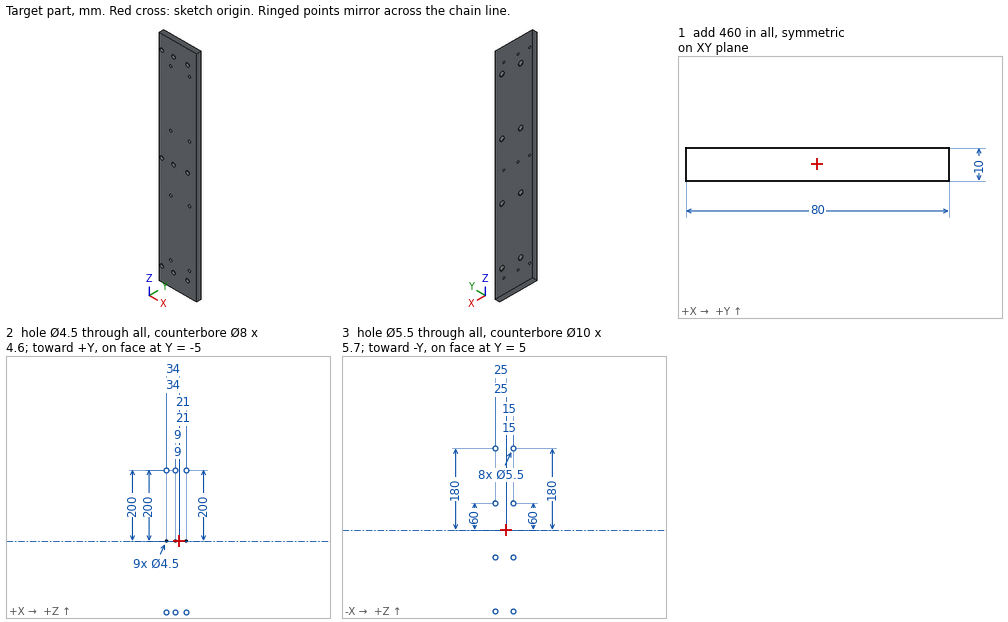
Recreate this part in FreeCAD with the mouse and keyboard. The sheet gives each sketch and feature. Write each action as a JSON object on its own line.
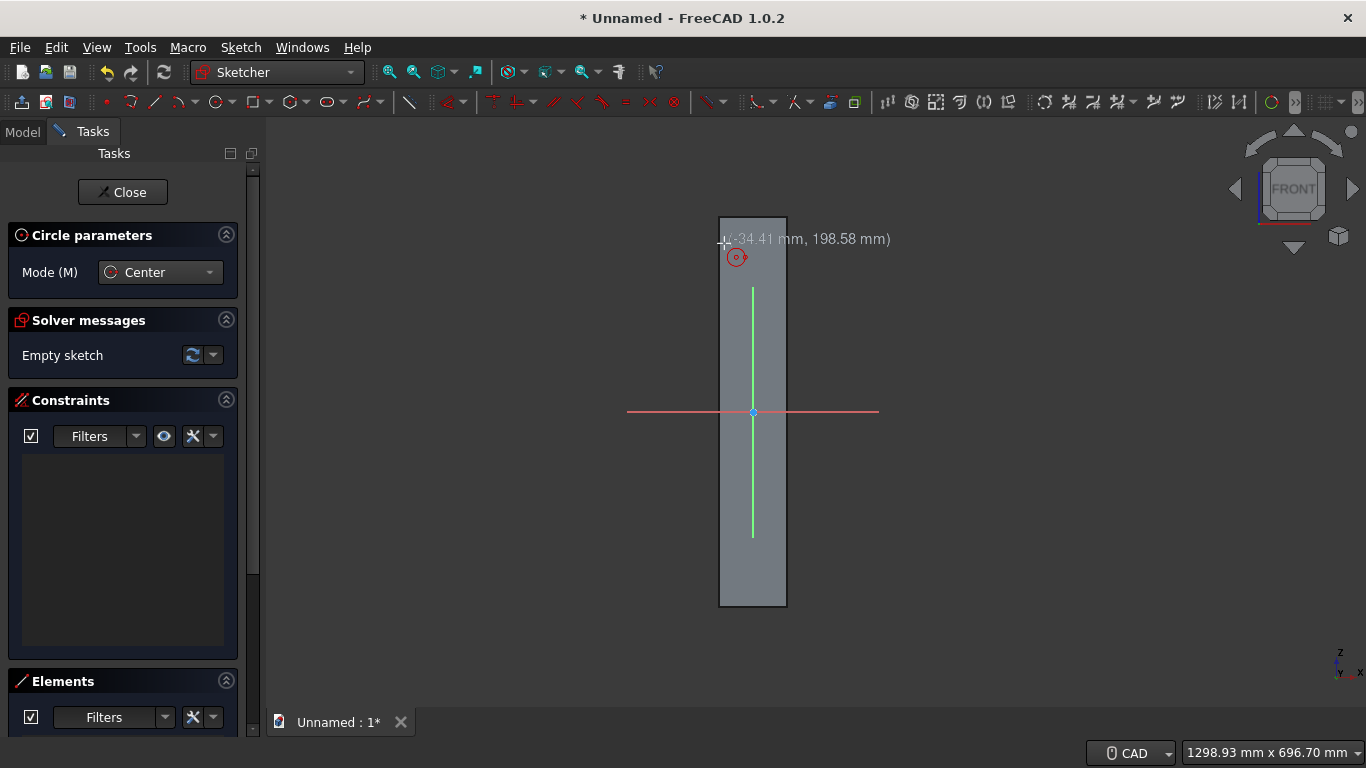
{"action": "left_click", "coordinate": [724, 243]}
{"action": "mouse_move", "coordinate": [726, 241]}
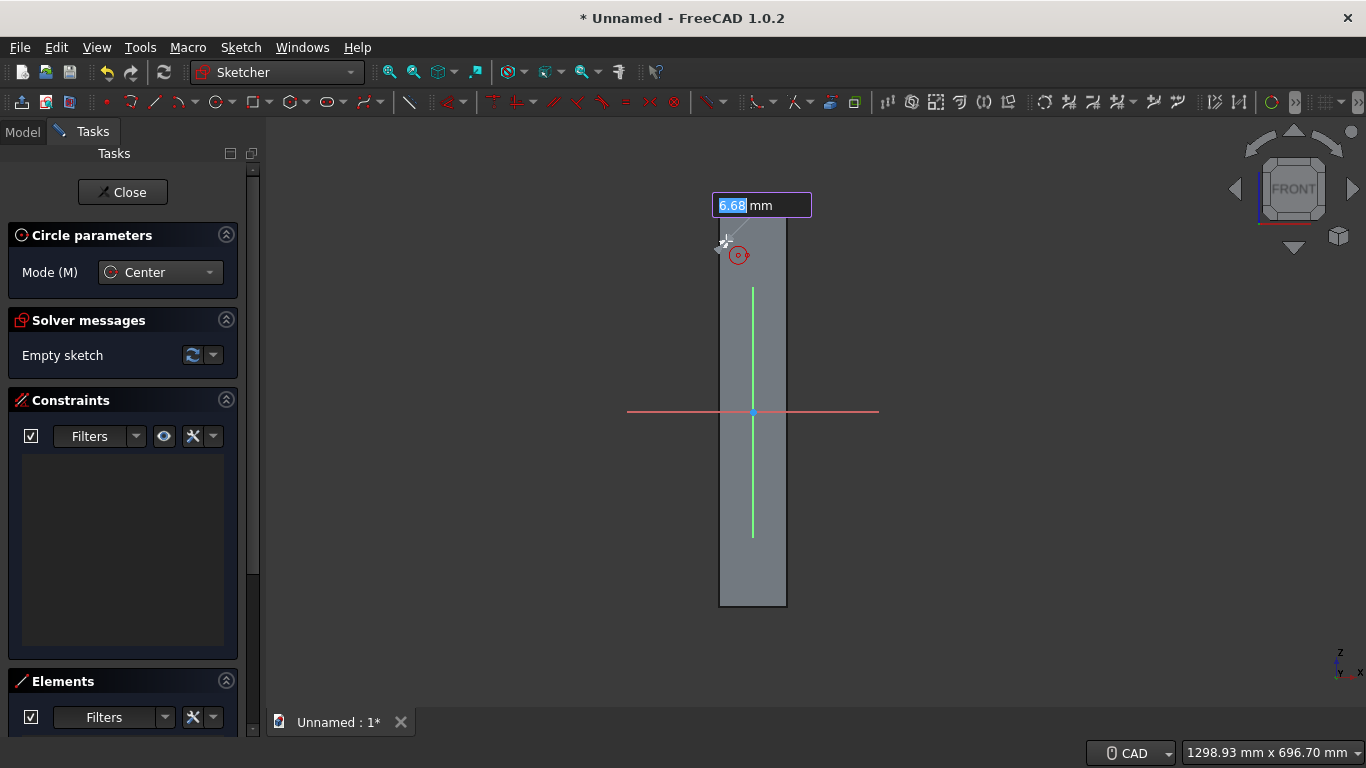
{"action": "type", "text": "4.5"}
{"action": "key", "text": "Return"}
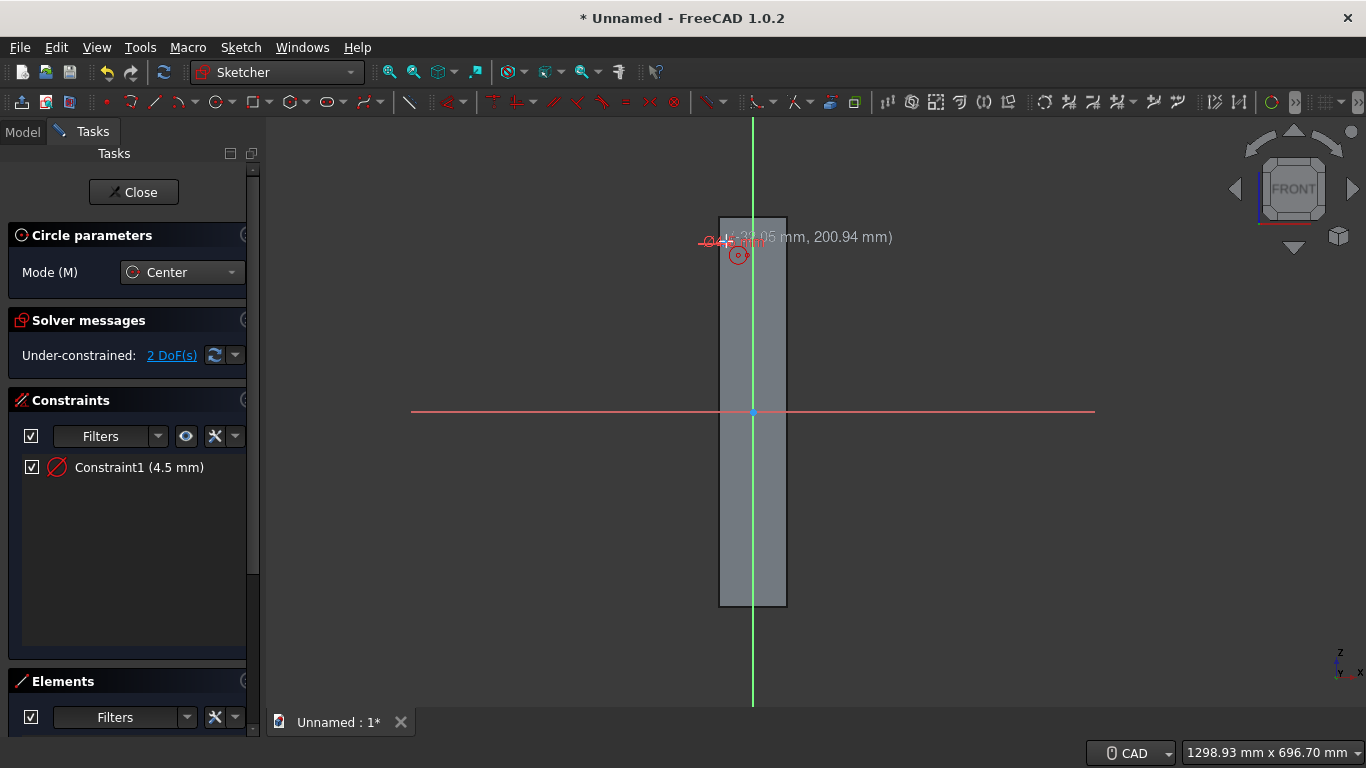
{"action": "scroll", "coordinate": [746, 243], "scroll_direction": "up", "scroll_amount": 13}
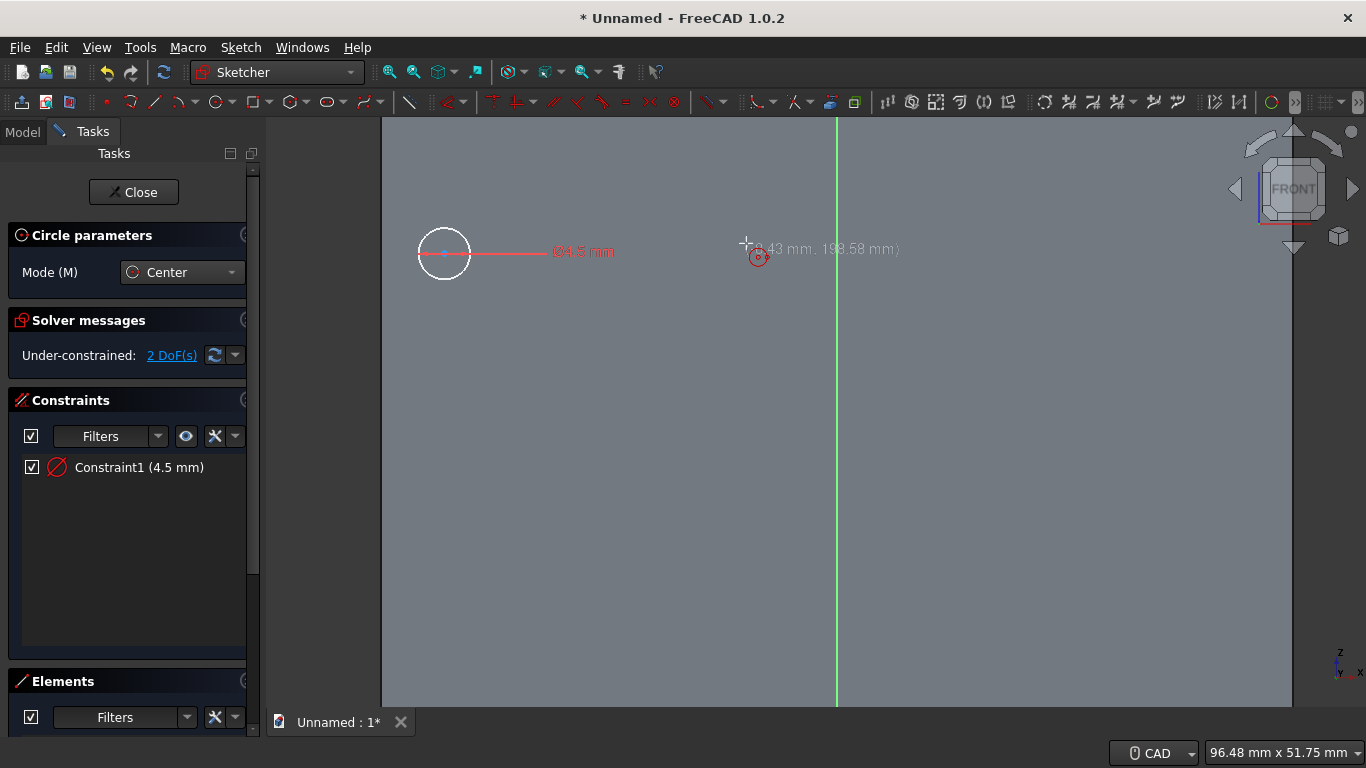
{"action": "scroll", "coordinate": [746, 243], "scroll_direction": "down", "scroll_amount": 13}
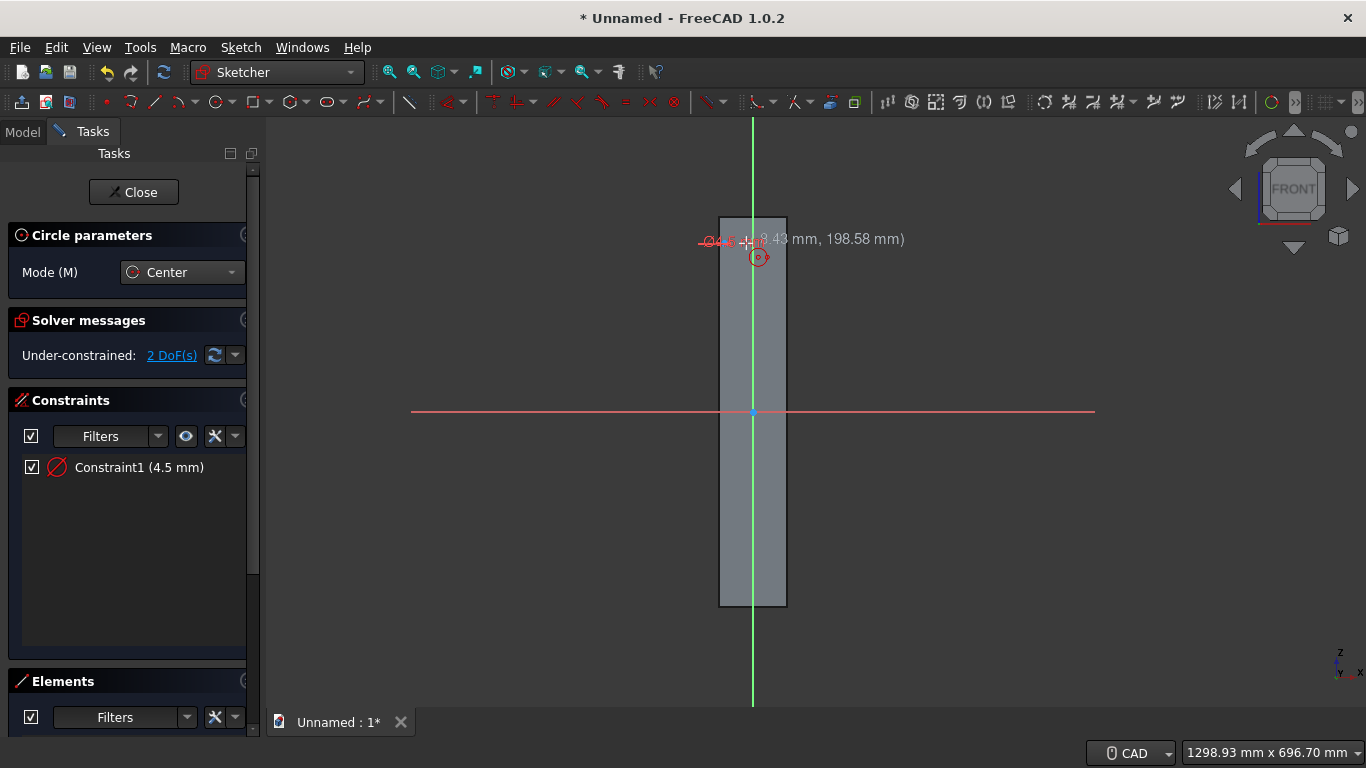
{"action": "scroll", "coordinate": [746, 243], "scroll_direction": "up", "scroll_amount": 4}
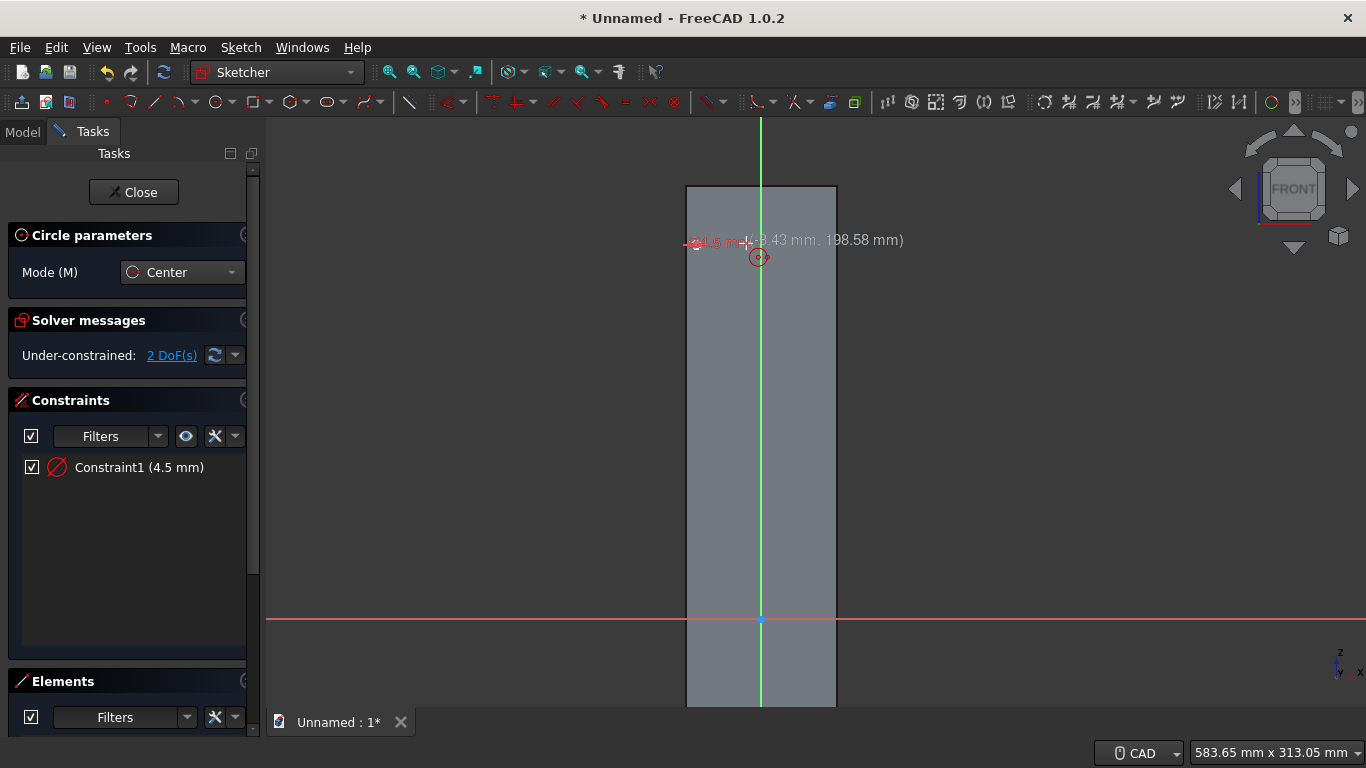
{"action": "left_click", "coordinate": [744, 242]}
{"action": "mouse_move", "coordinate": [741, 239]}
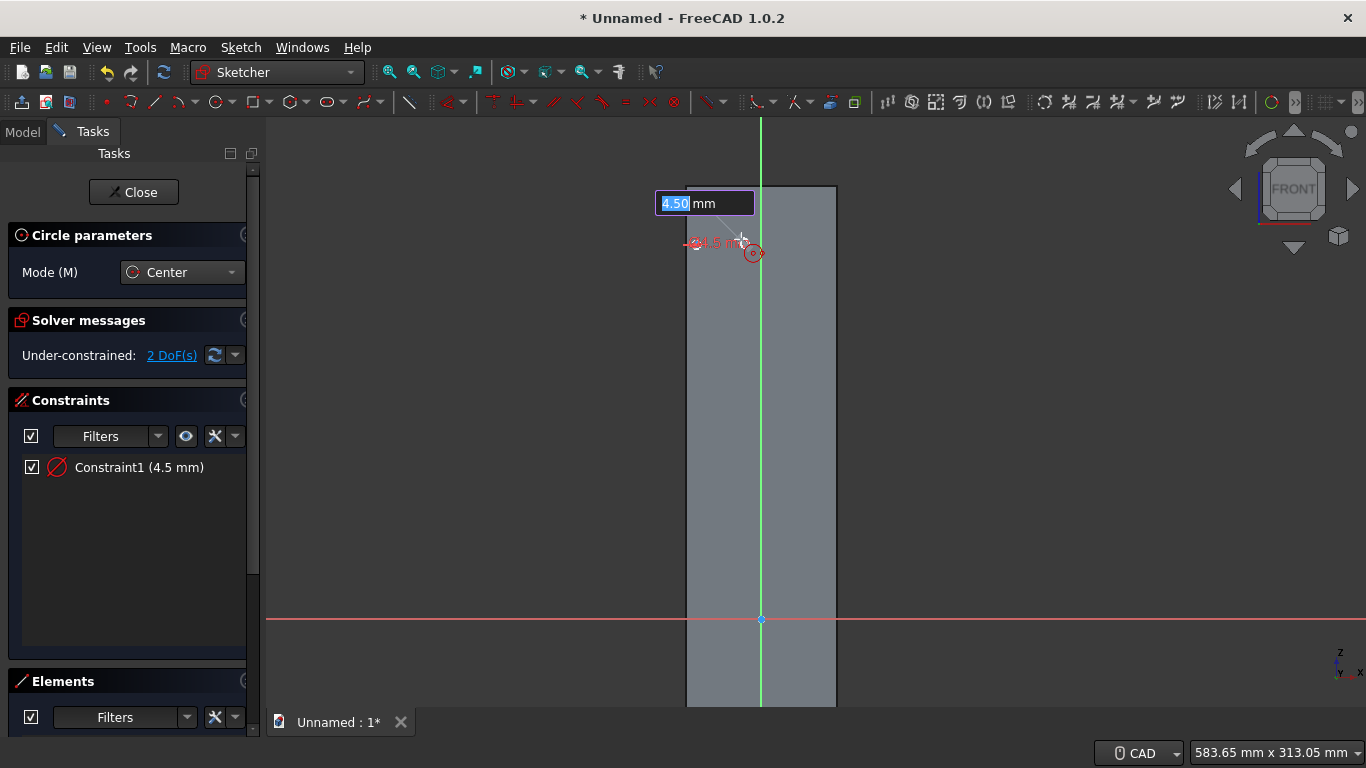
{"action": "type", "text": "4.5"}
{"action": "key", "text": "Return"}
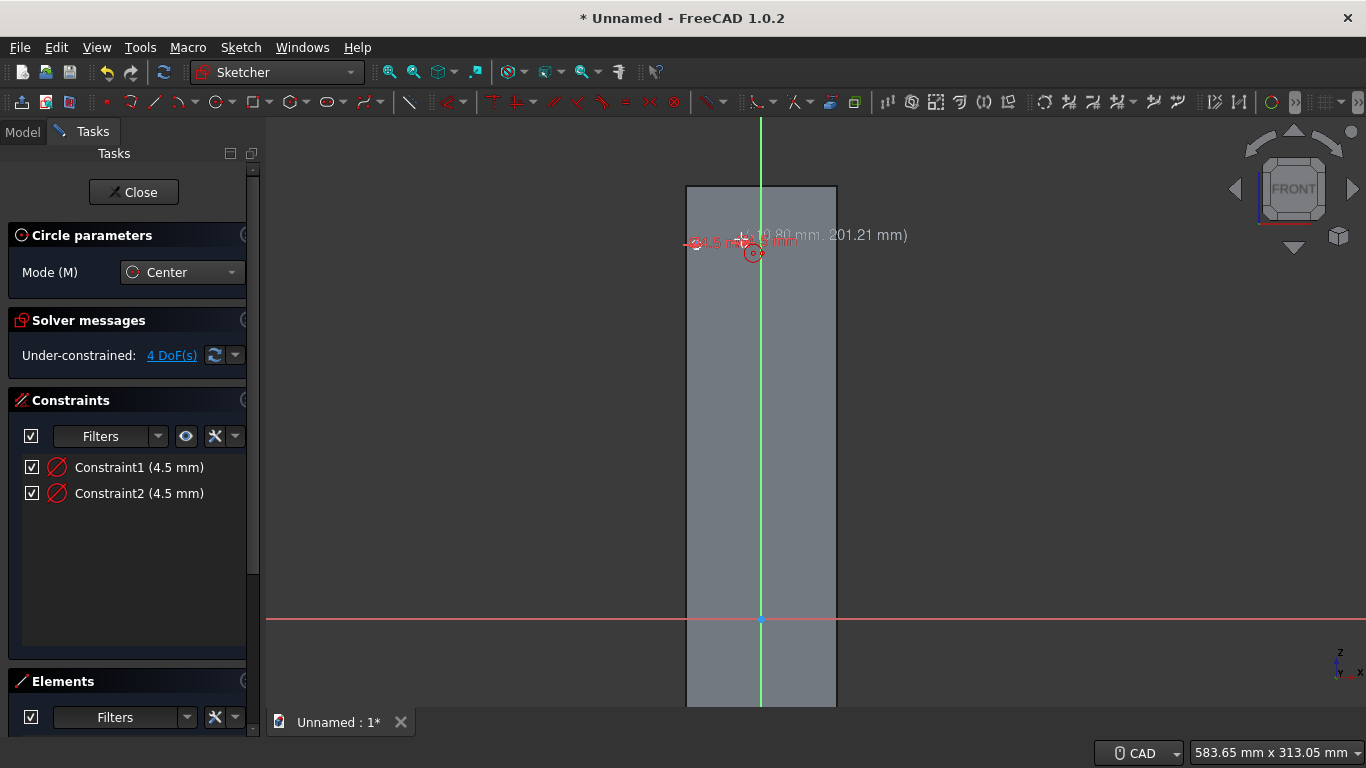
{"action": "scroll", "coordinate": [801, 242], "scroll_direction": "up", "scroll_amount": 9}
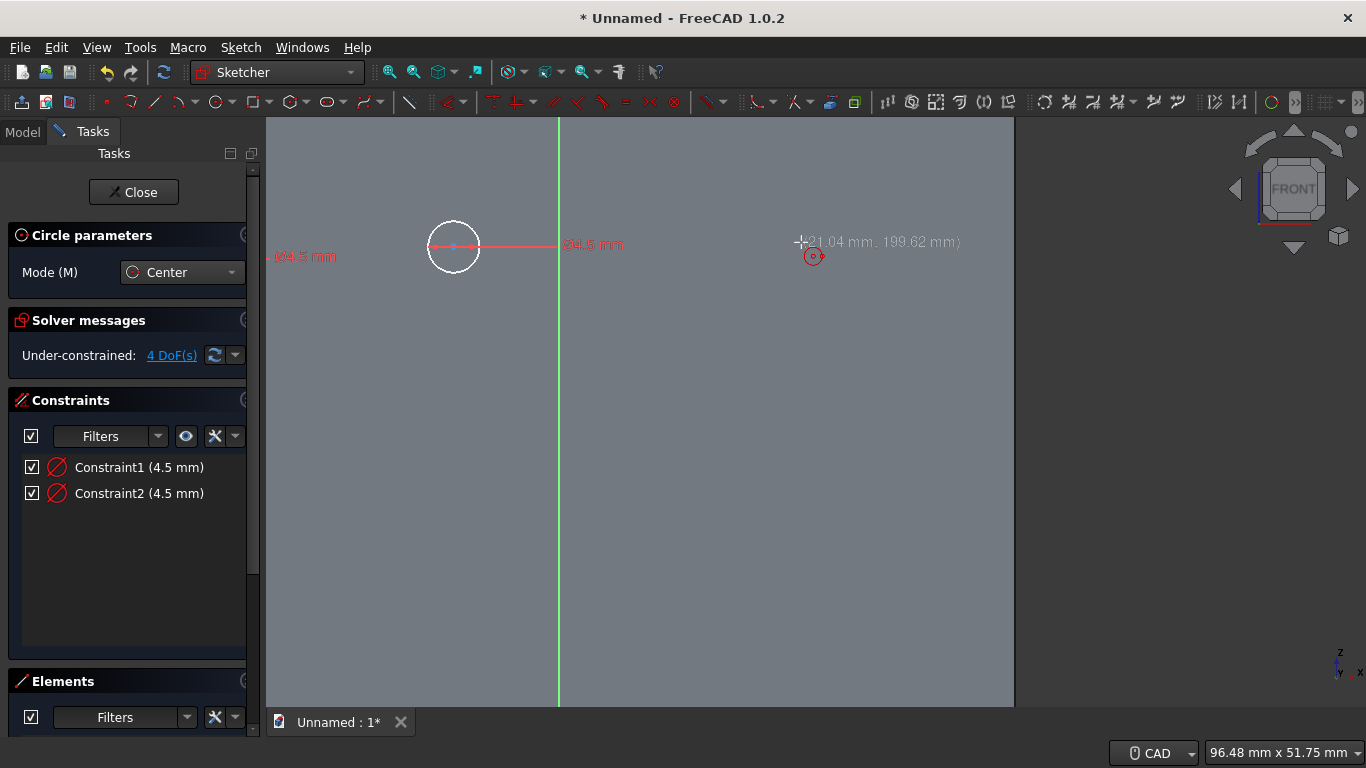
{"action": "scroll", "coordinate": [769, 243], "scroll_direction": "down", "scroll_amount": 13}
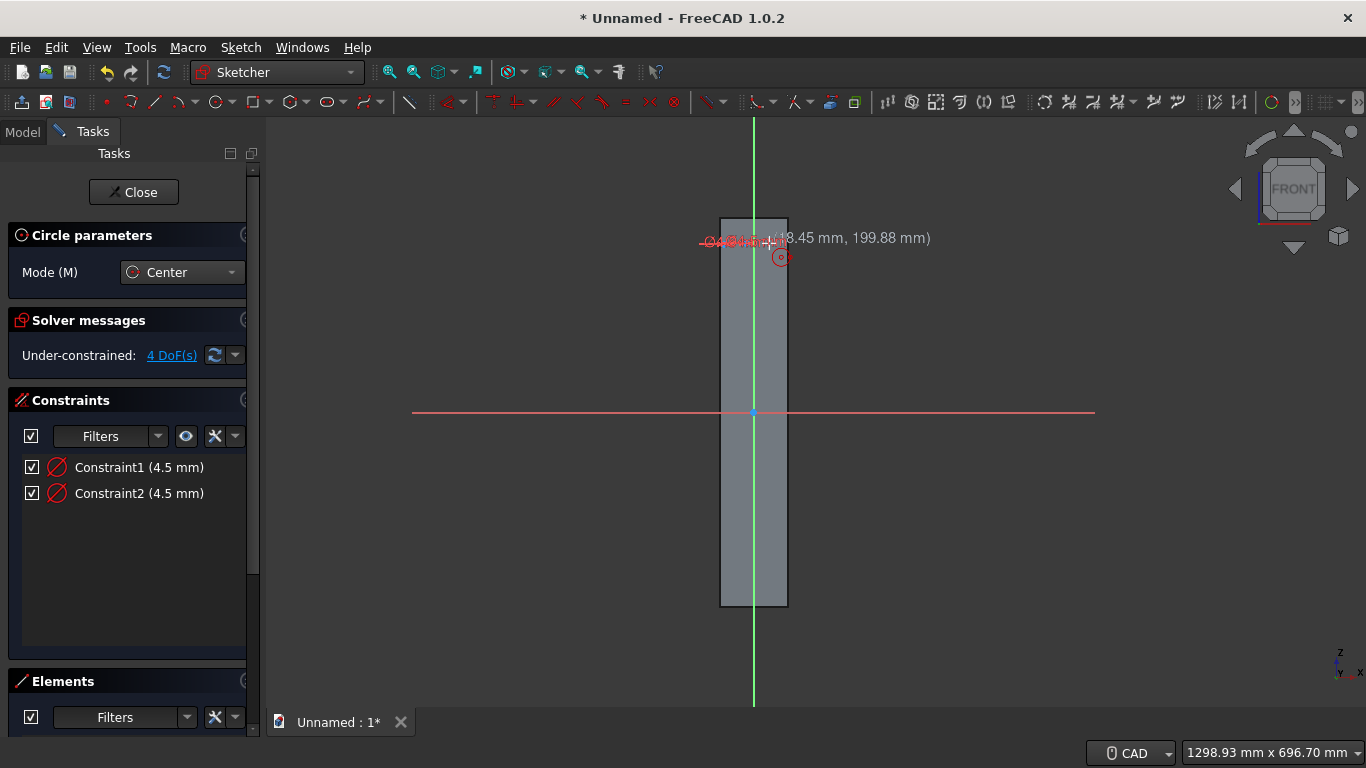
{"action": "left_click", "coordinate": [772, 243]}
{"action": "mouse_move", "coordinate": [773, 242]}